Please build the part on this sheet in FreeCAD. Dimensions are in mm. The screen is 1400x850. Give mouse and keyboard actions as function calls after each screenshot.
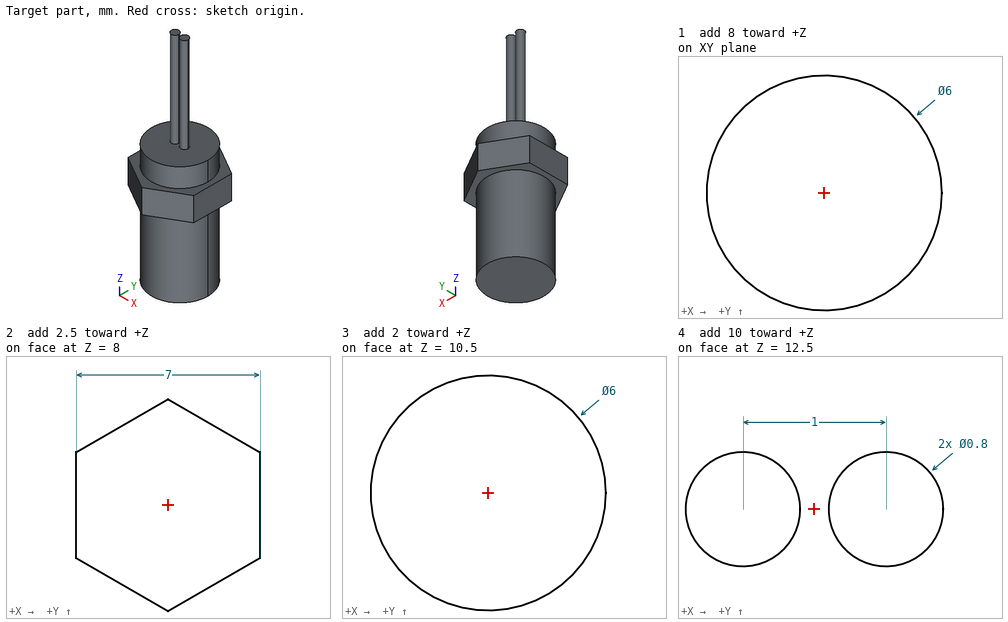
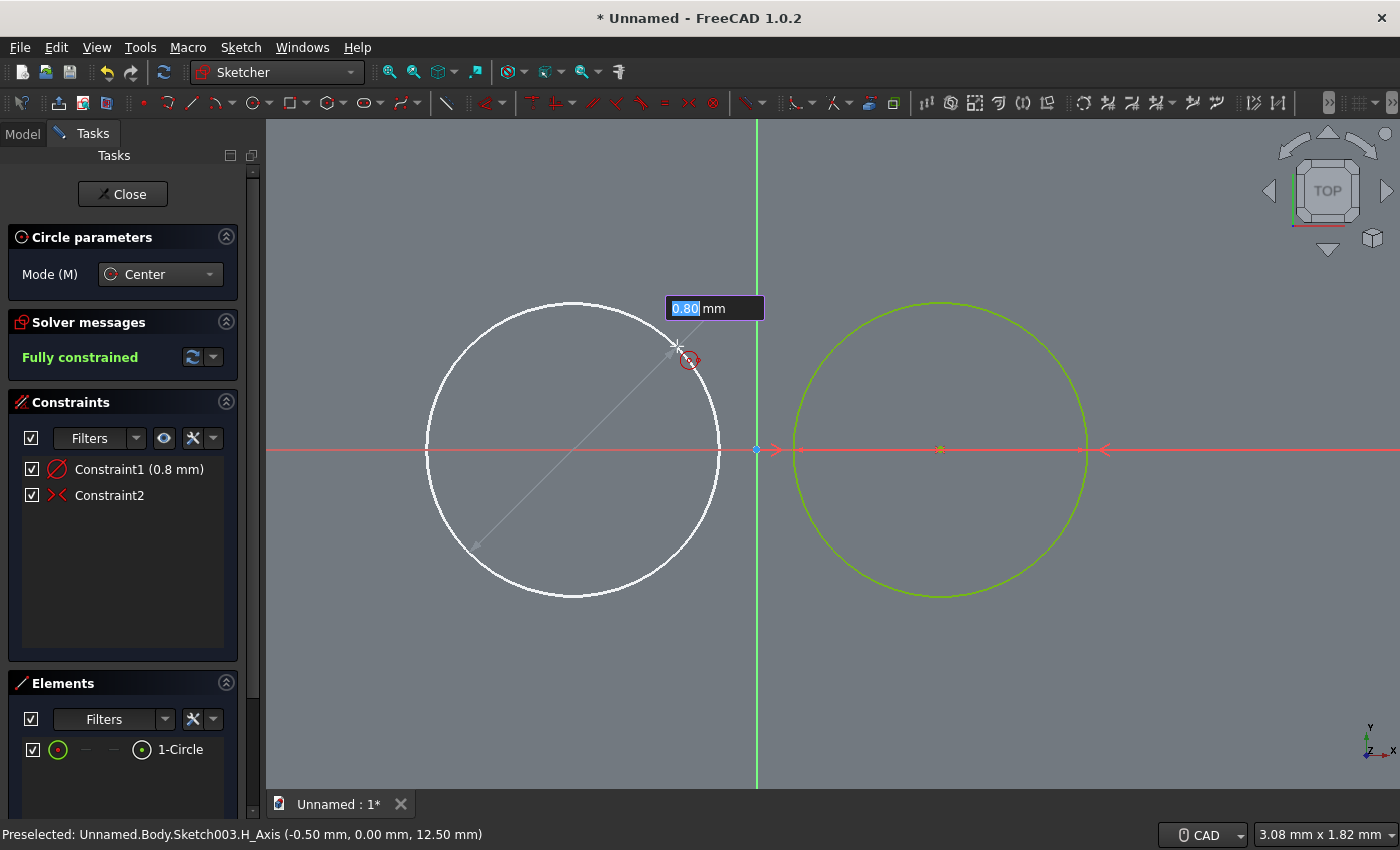
text(0.8)
key(Return)
key(Escape)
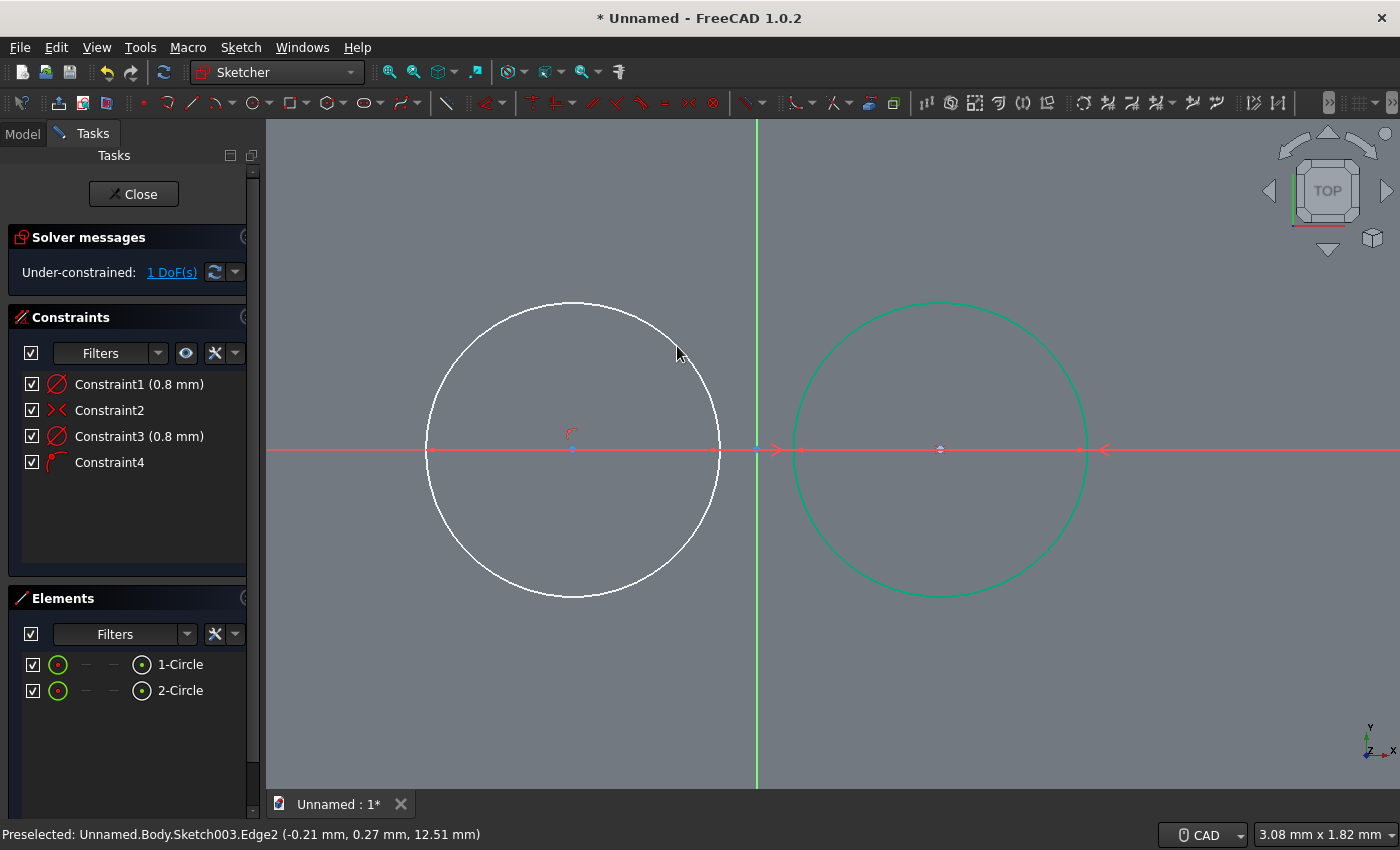
click(940, 450)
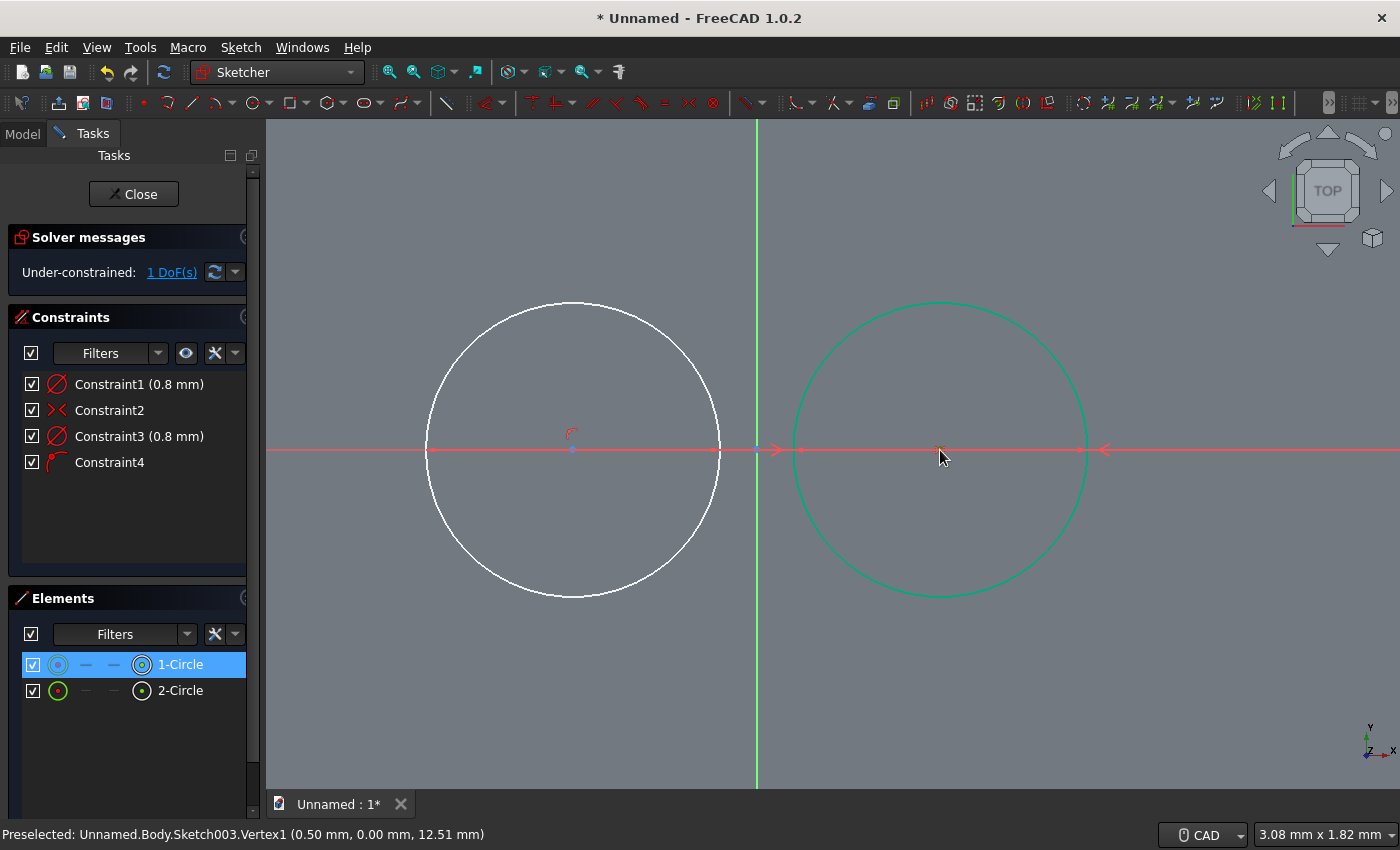
click(573, 450)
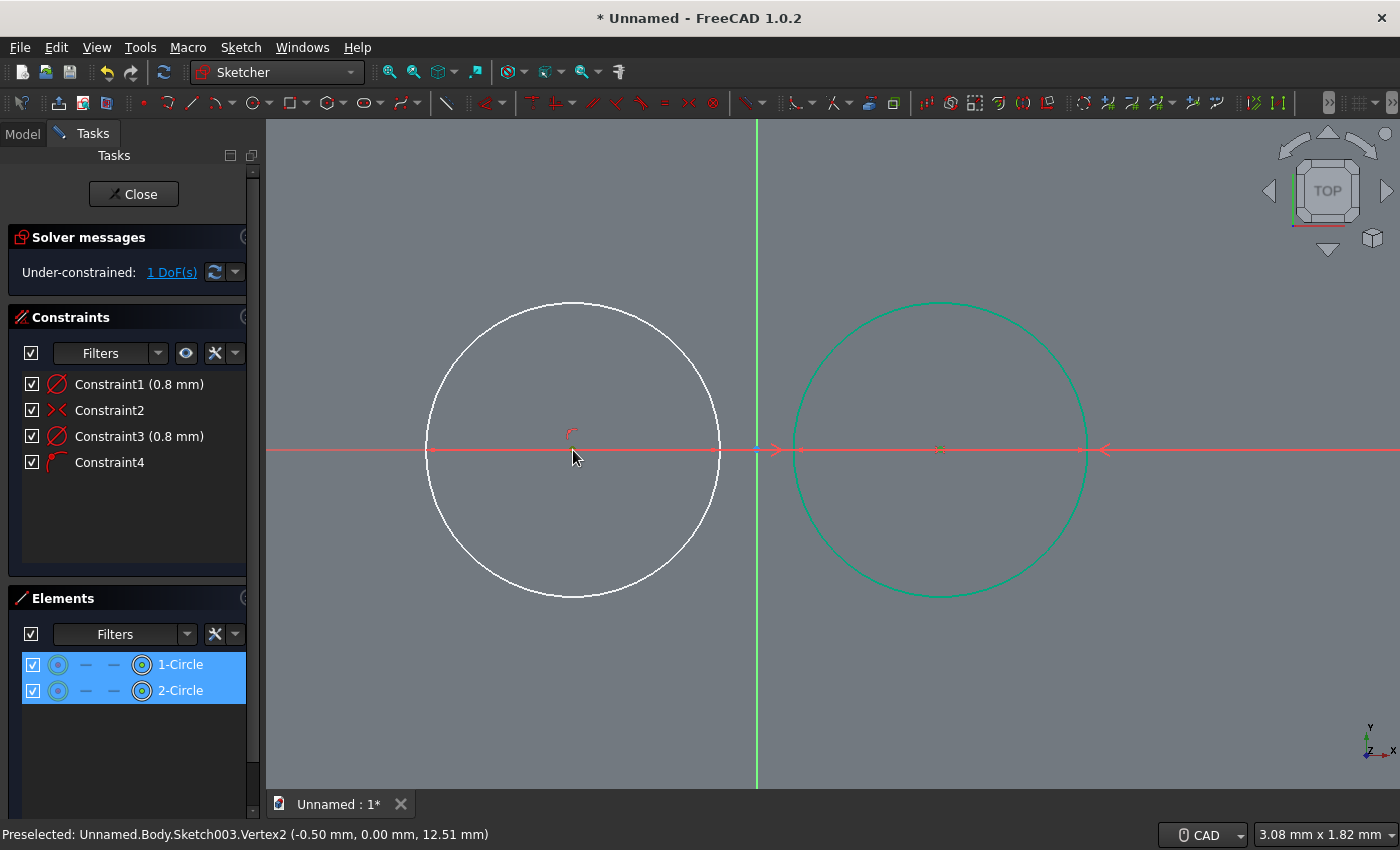
key(l)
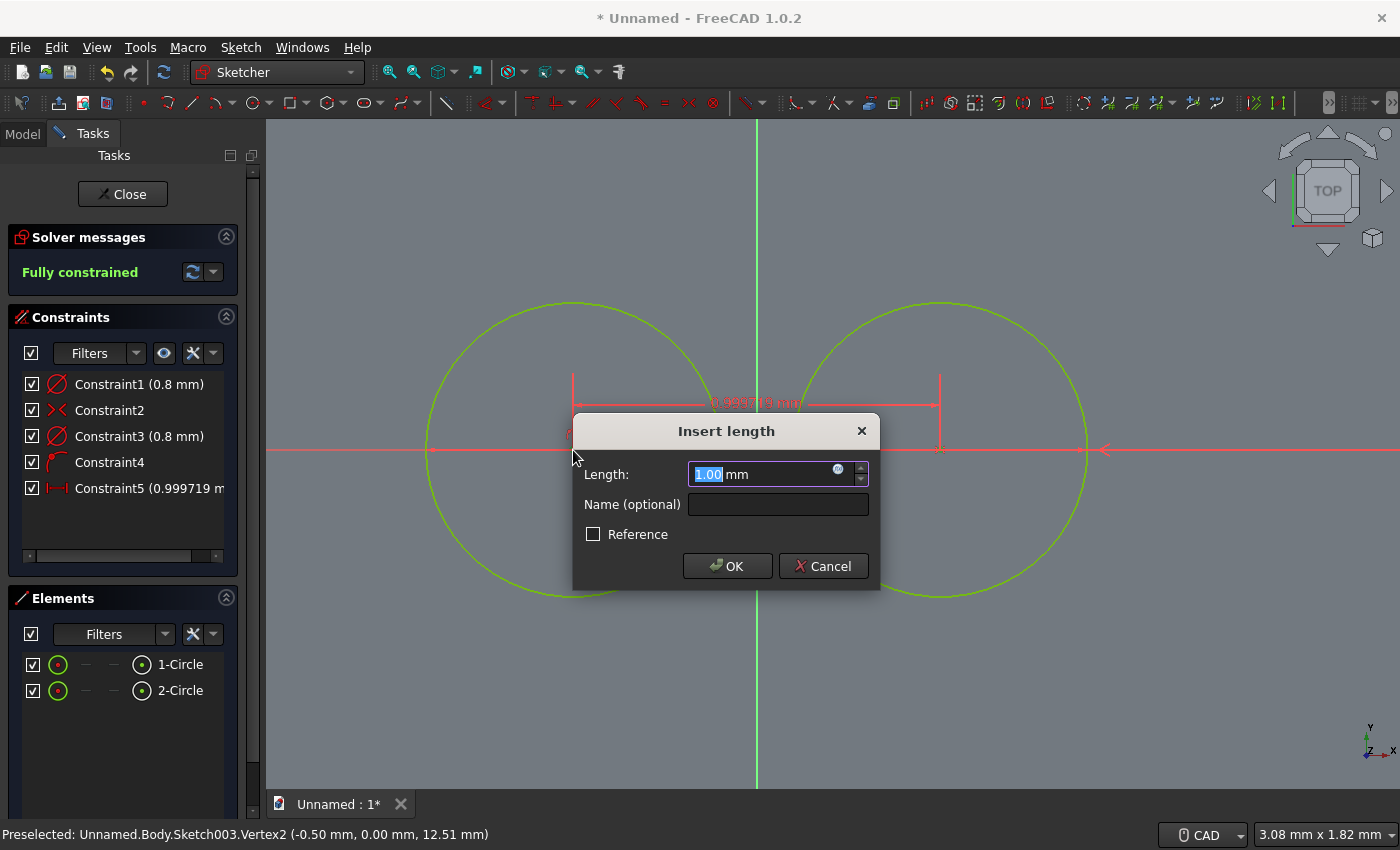
text(1)
key(Return)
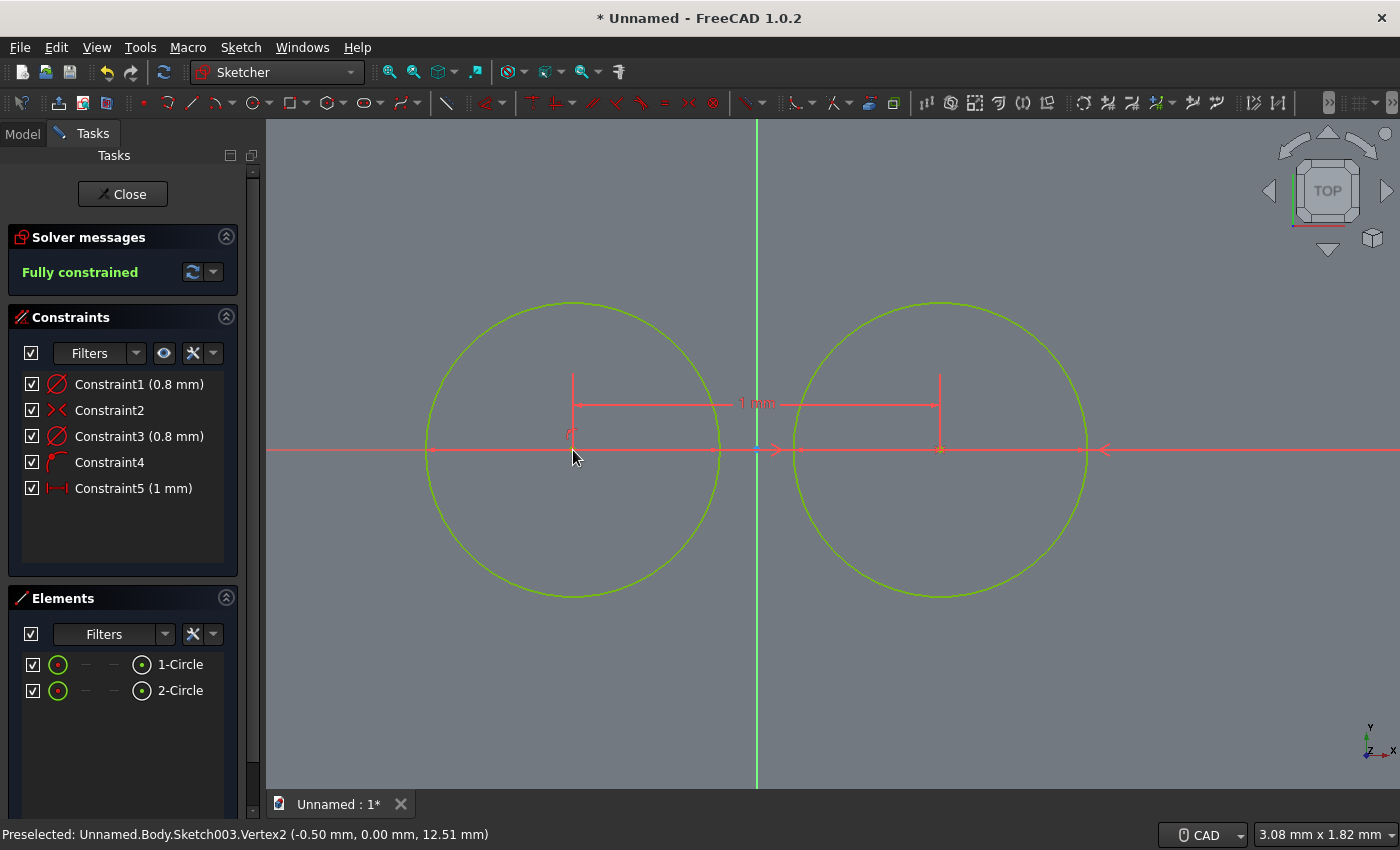
click(123, 194)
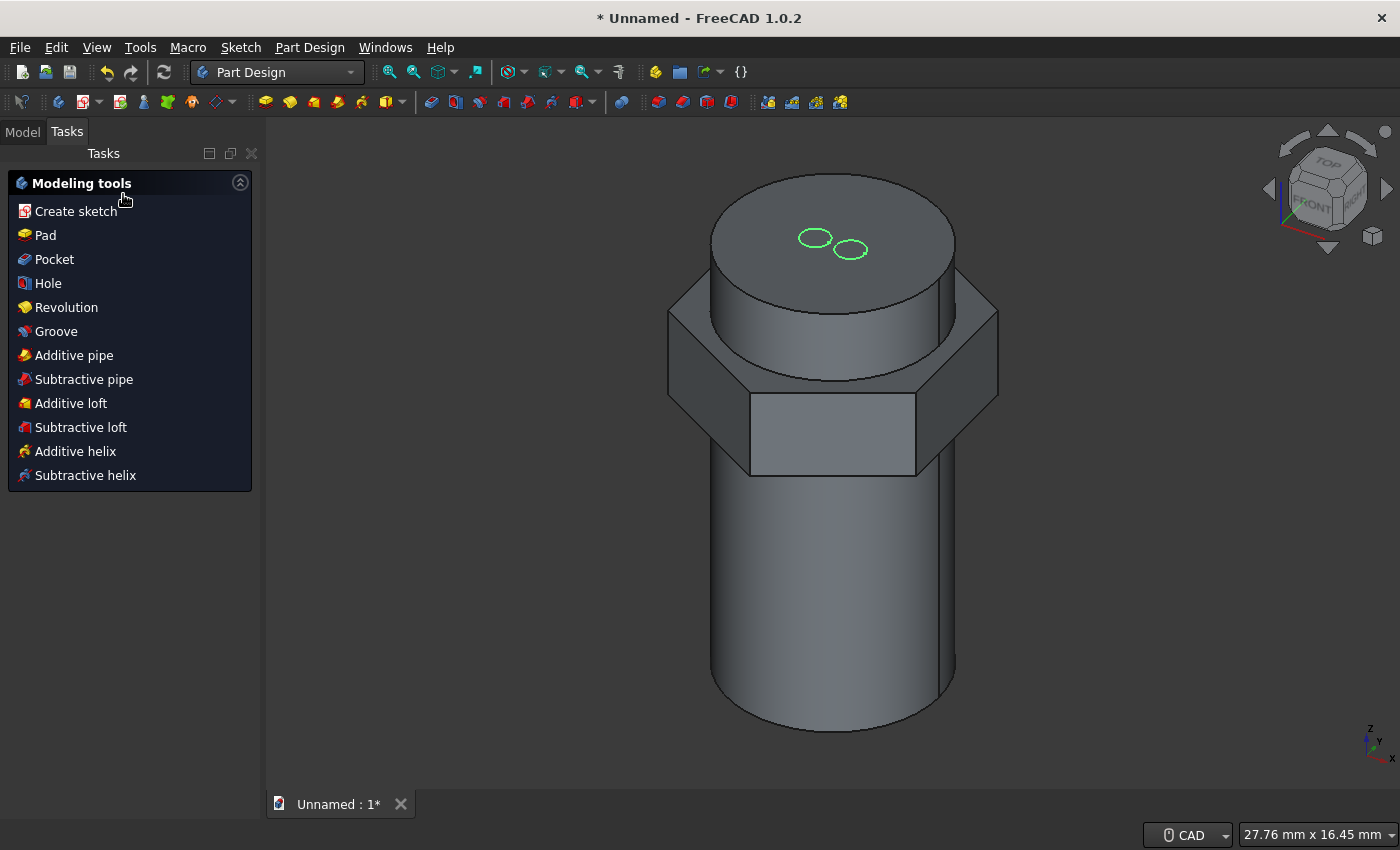
click(266, 102)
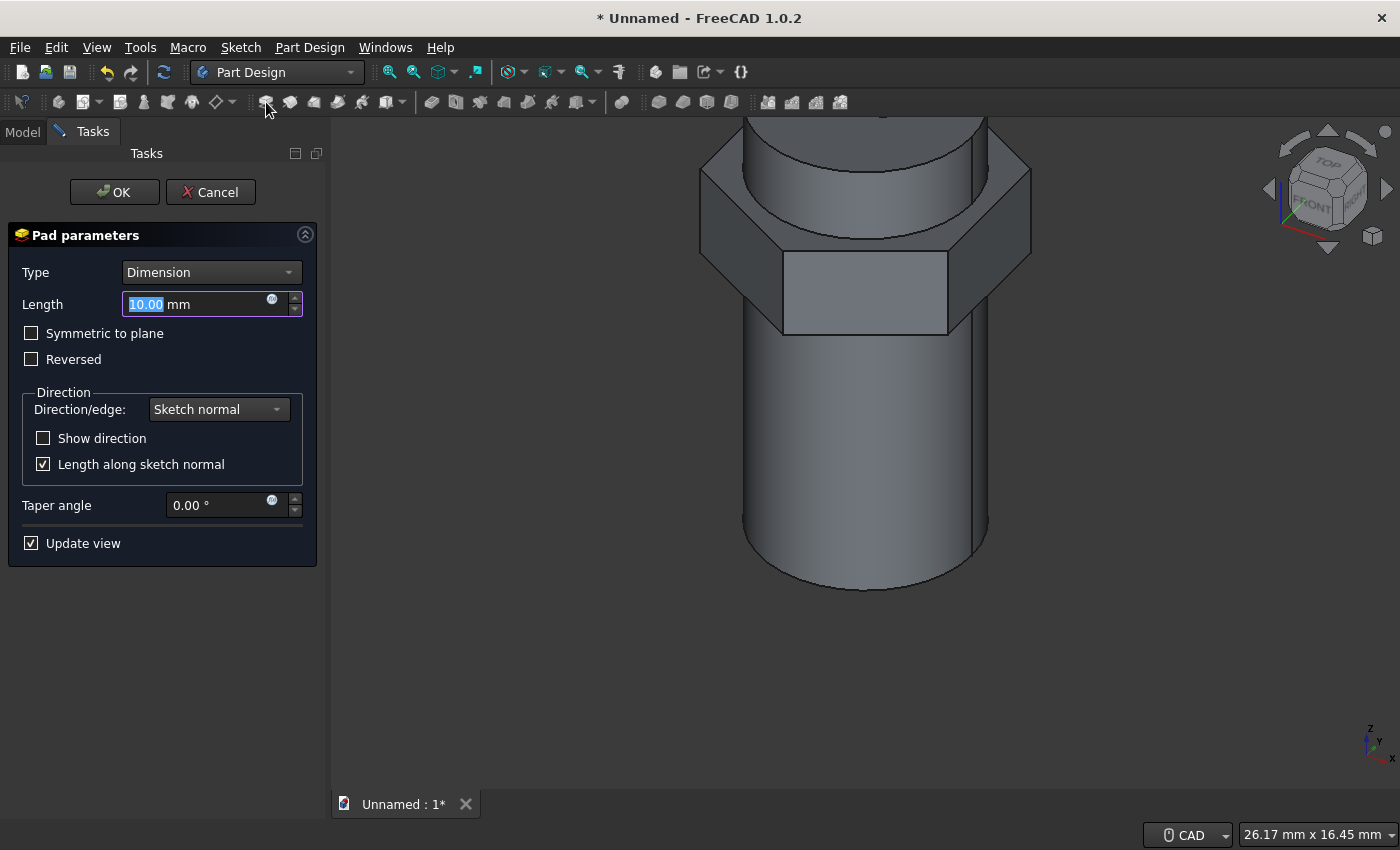
text(10)
key(Tab)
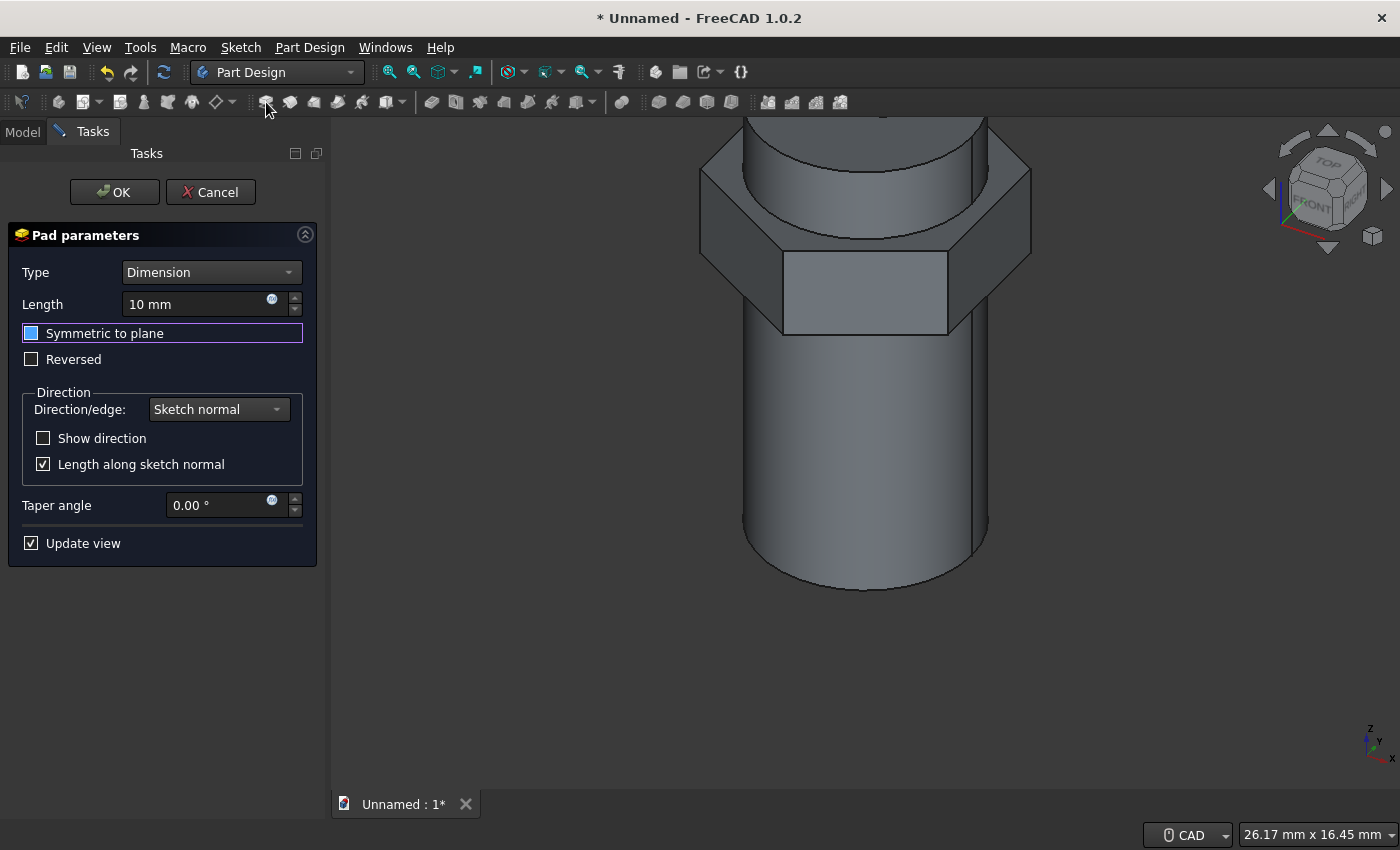
click(115, 192)